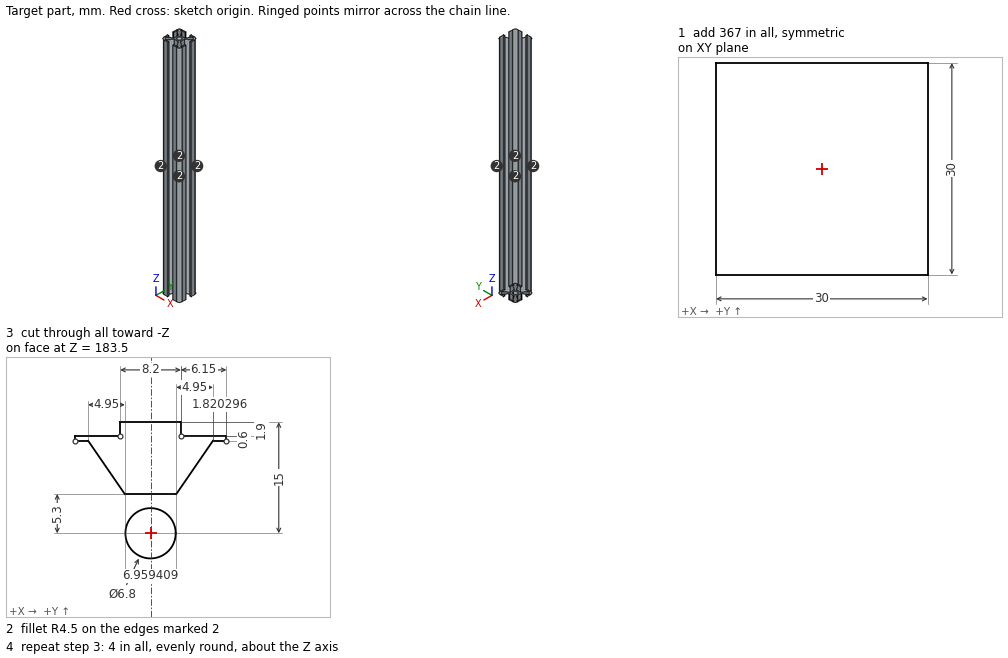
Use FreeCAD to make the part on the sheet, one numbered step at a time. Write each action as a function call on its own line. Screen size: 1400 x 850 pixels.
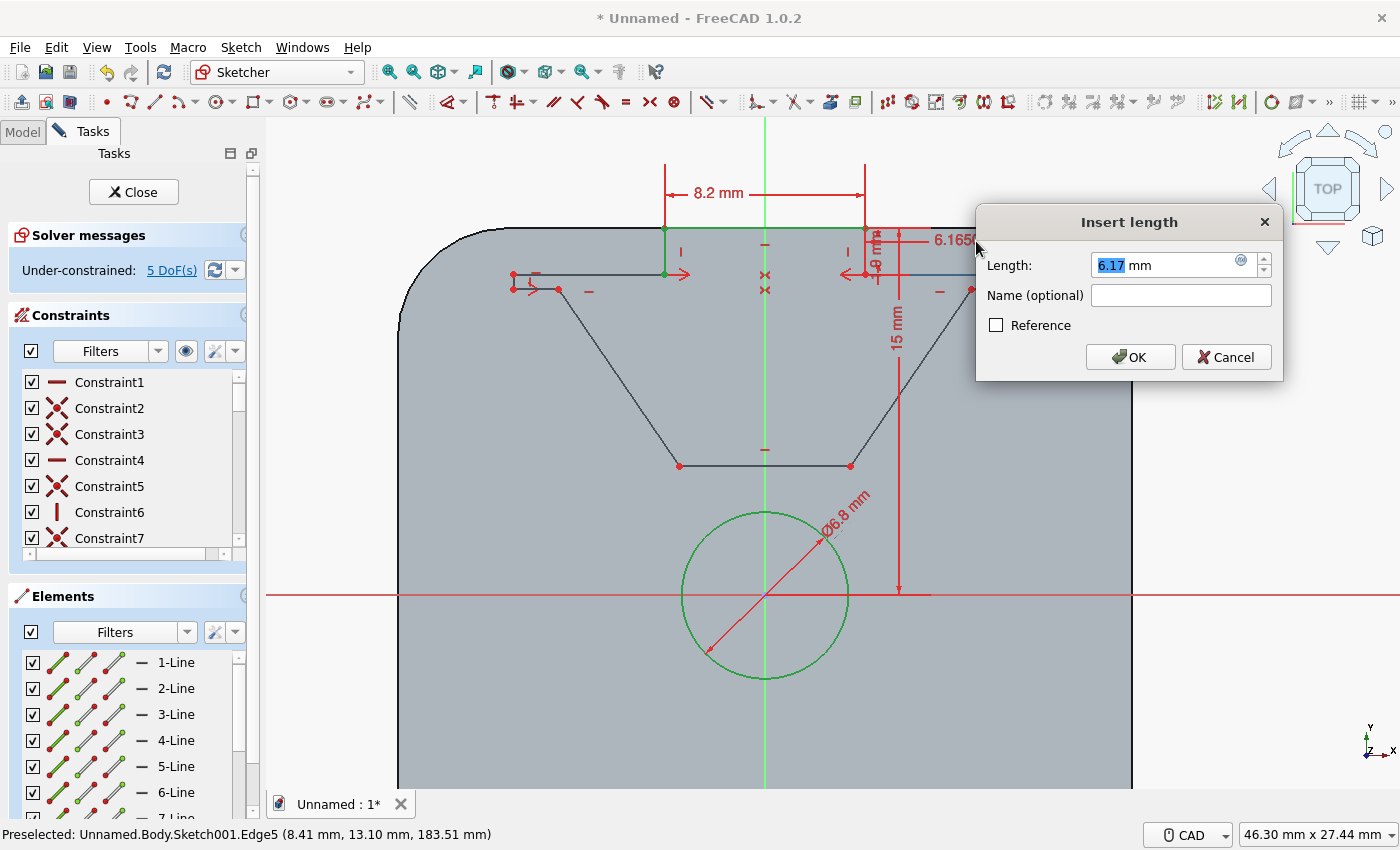
text(6.15)
key(Return)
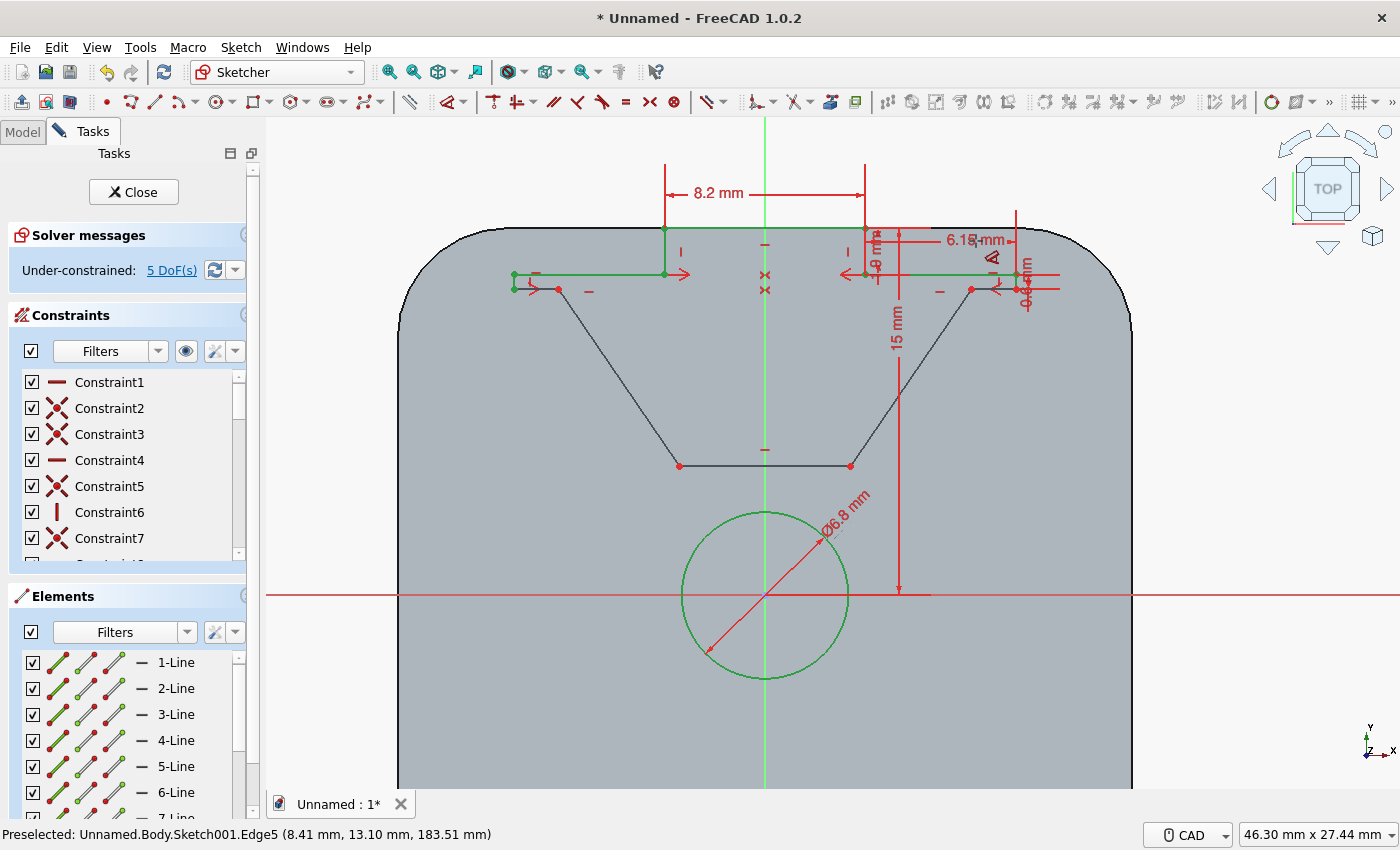
click(680, 466)
click(646, 531)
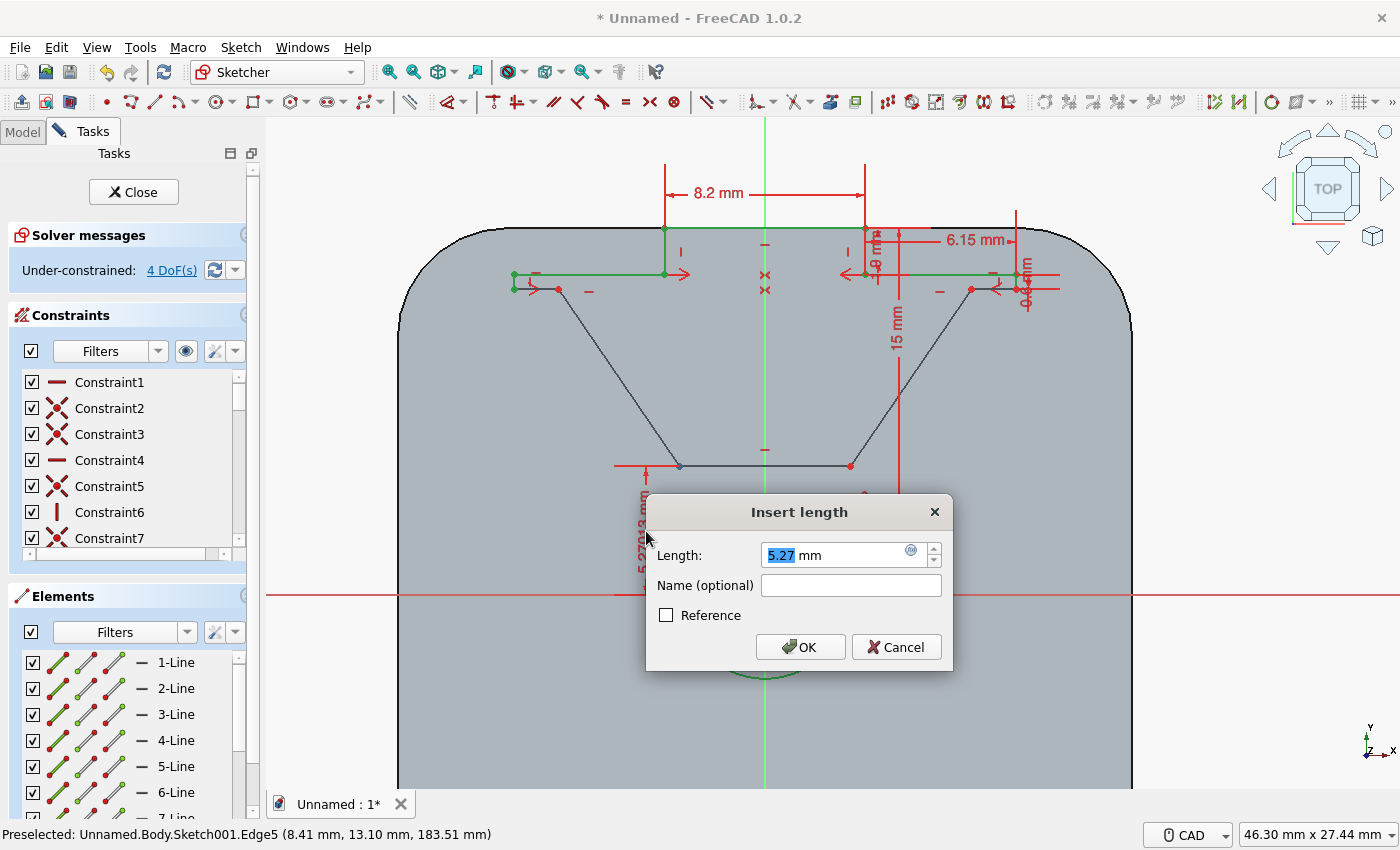
text(5.3)
key(Return)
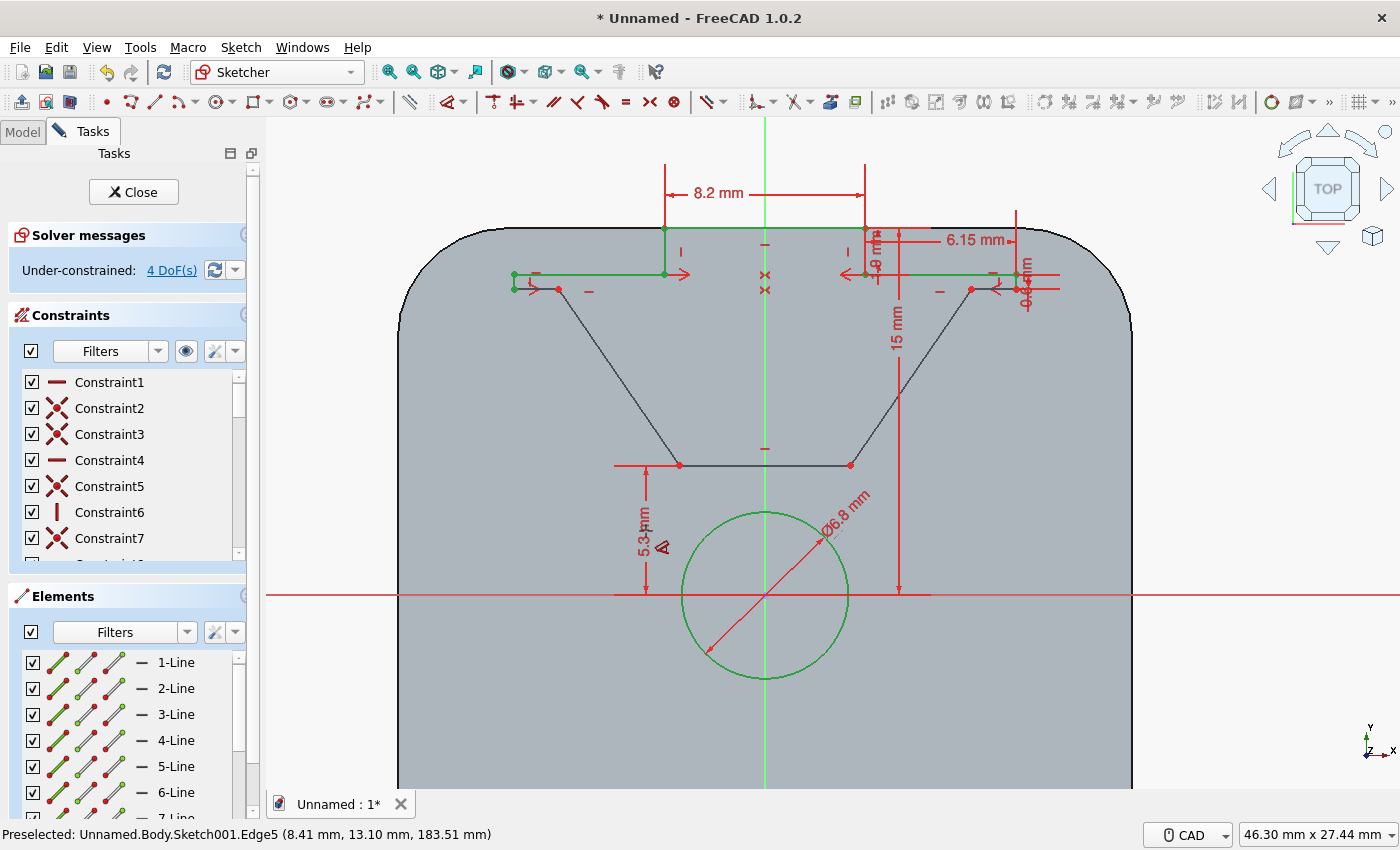
click(887, 413)
click(939, 500)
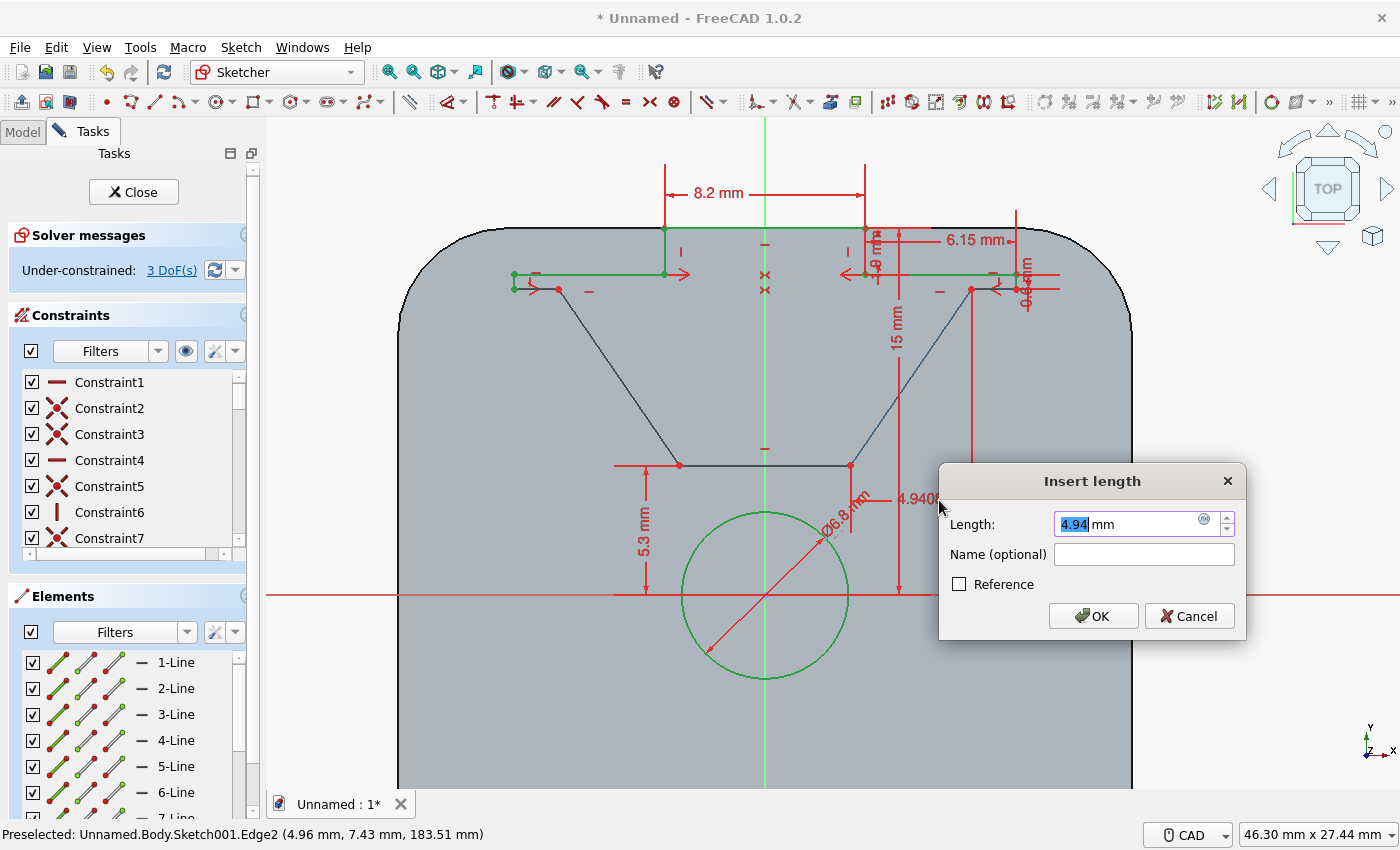
text(4.95)
key(Return)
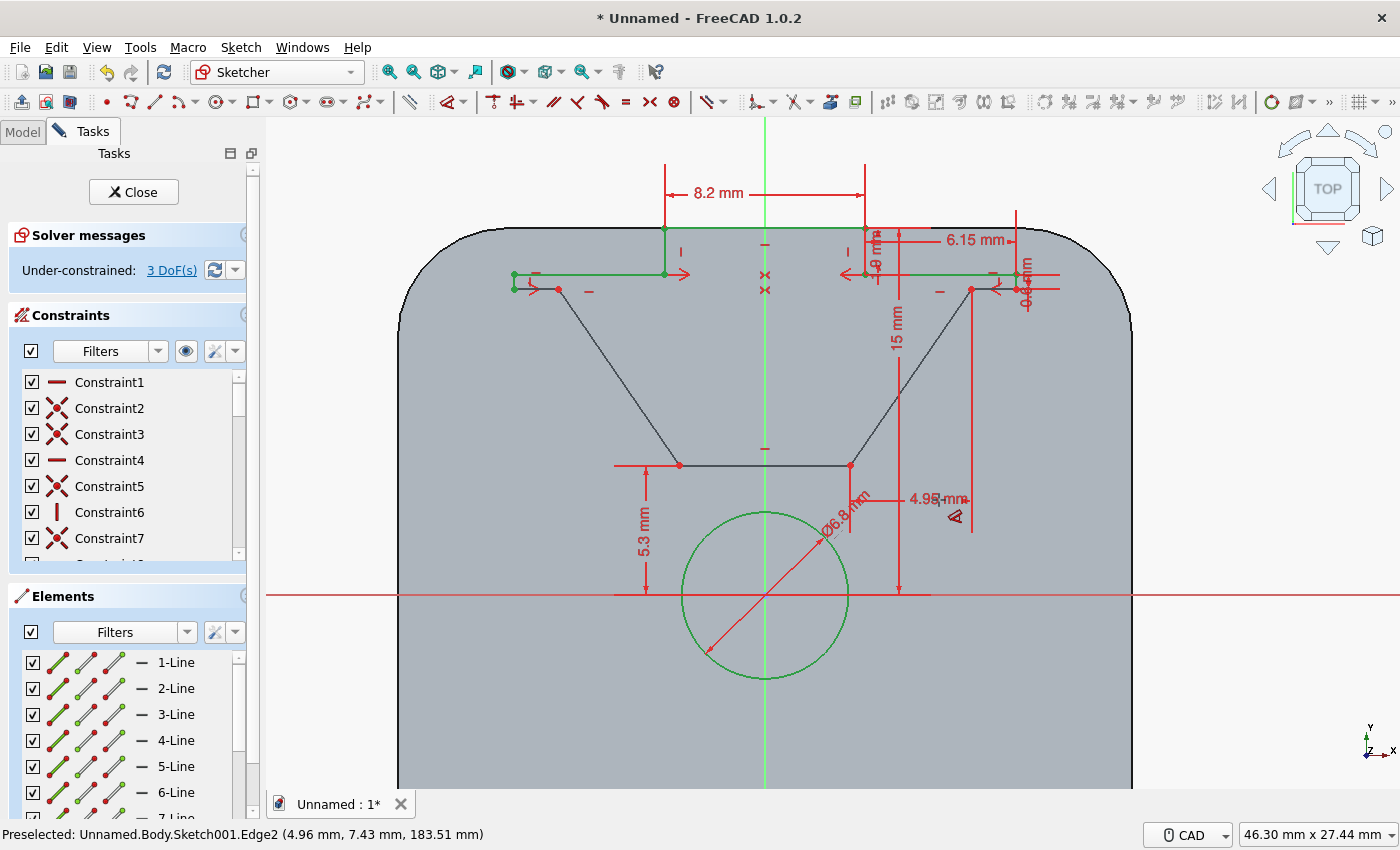
click(595, 342)
click(619, 255)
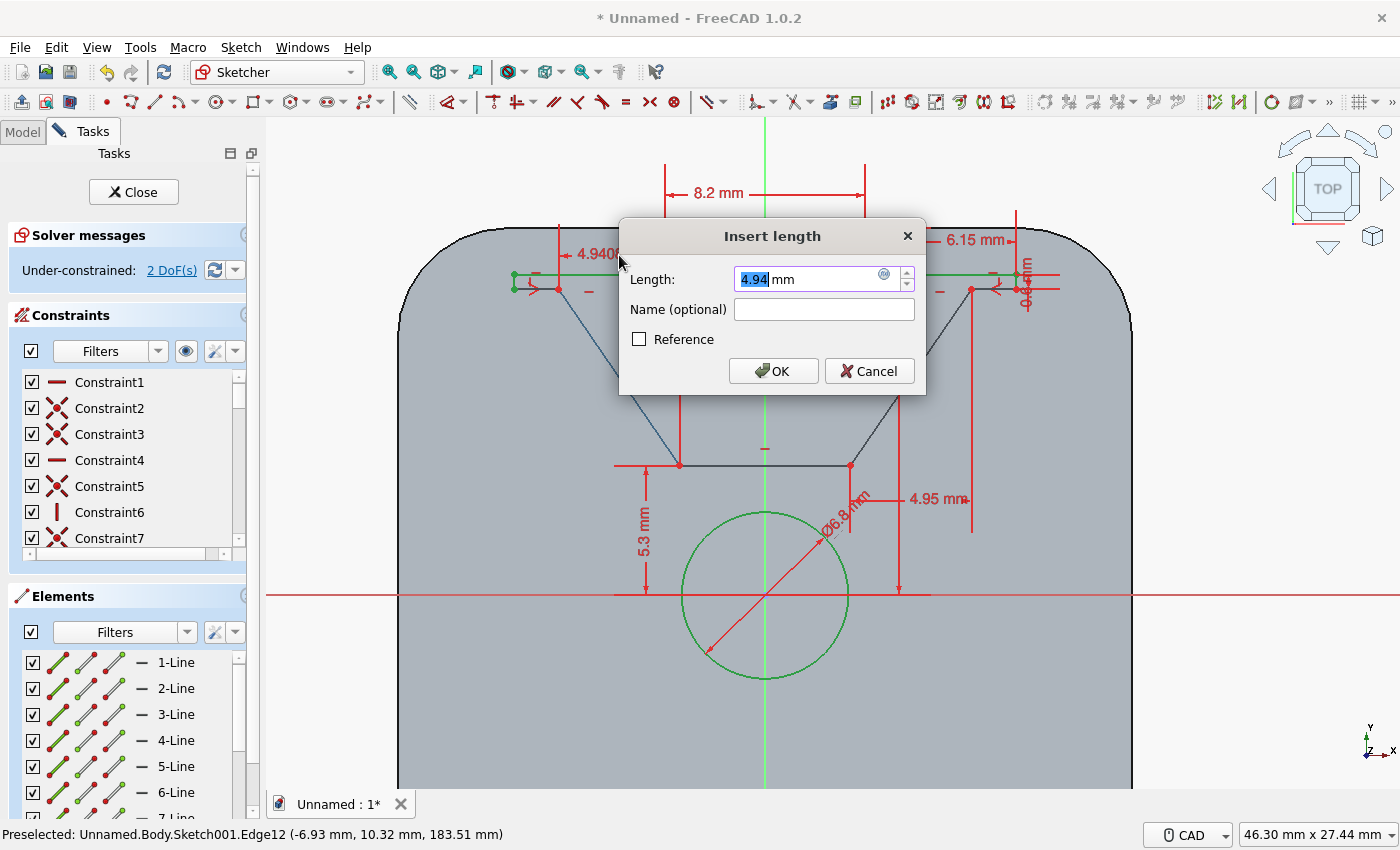
text(4.95)
key(Return)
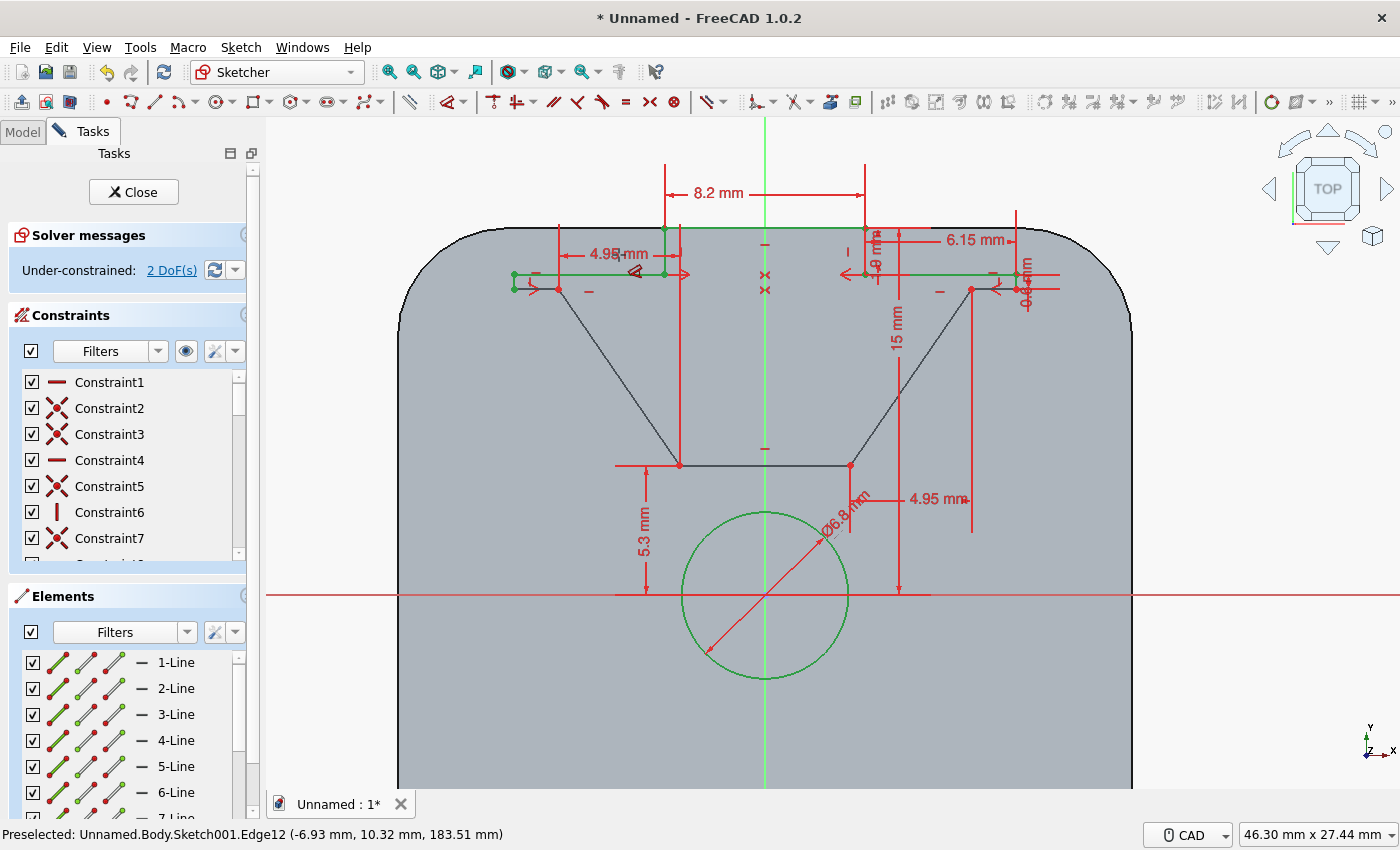
click(731, 466)
click(726, 500)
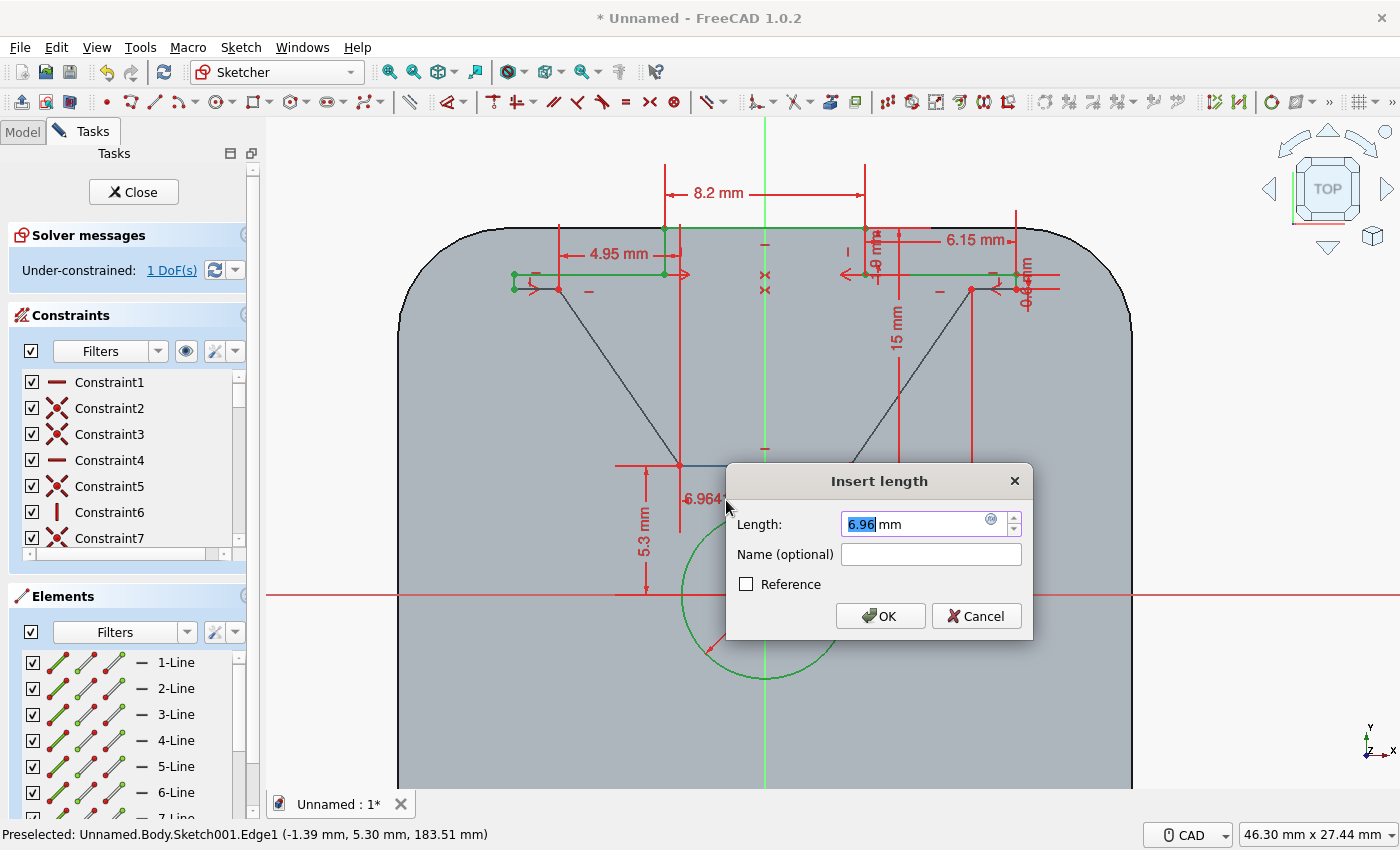
text(6.959409)
key(Return)